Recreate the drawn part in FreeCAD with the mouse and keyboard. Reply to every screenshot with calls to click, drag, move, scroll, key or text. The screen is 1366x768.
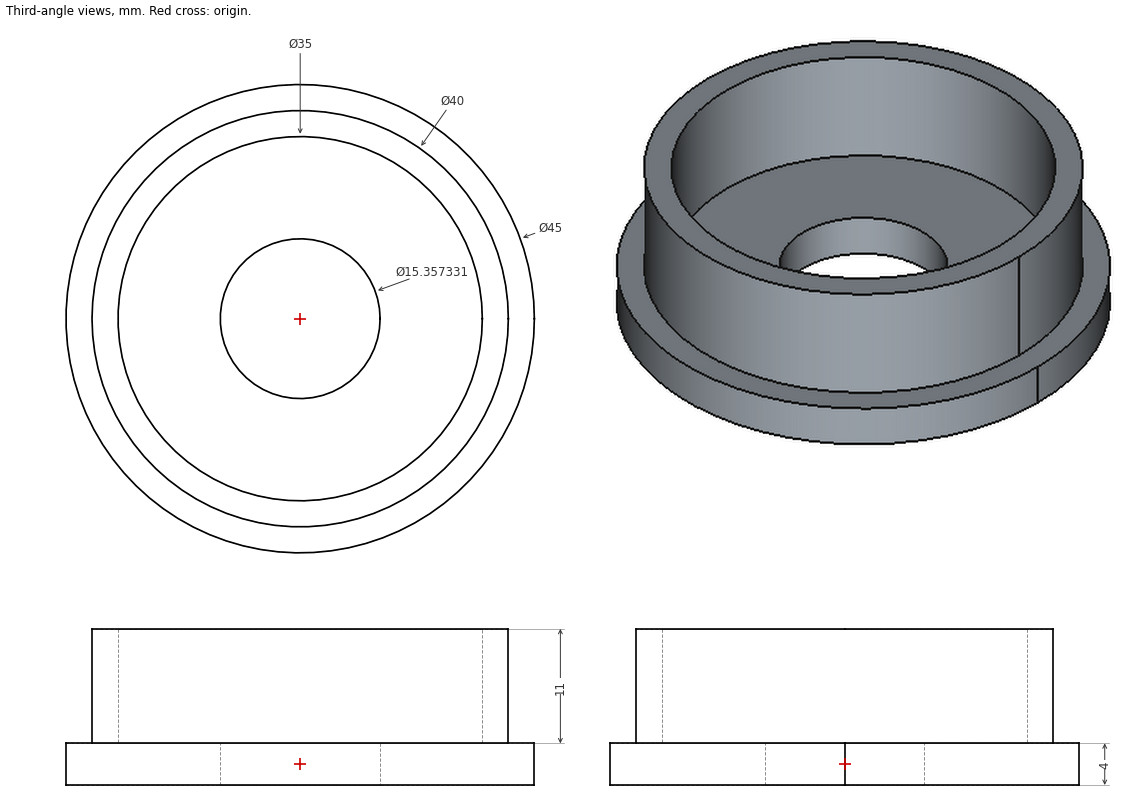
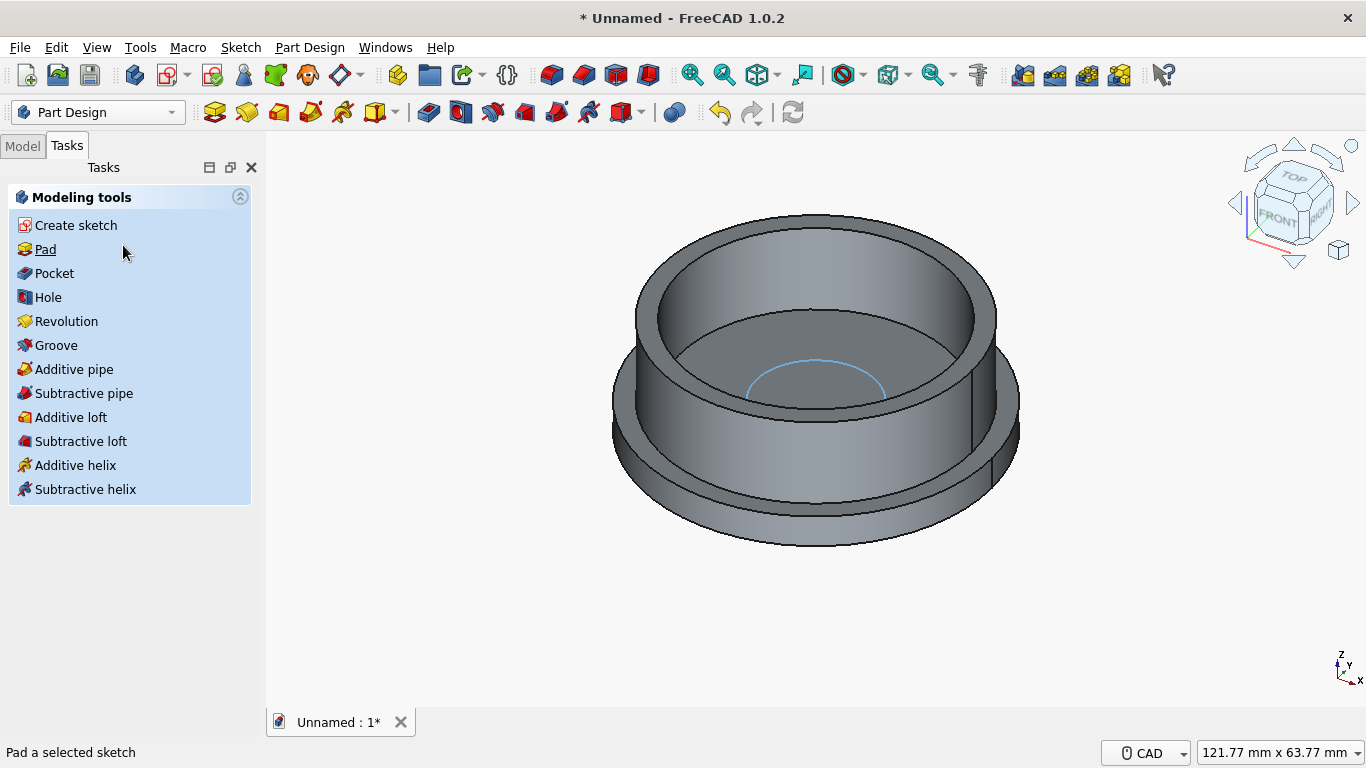
click(430, 112)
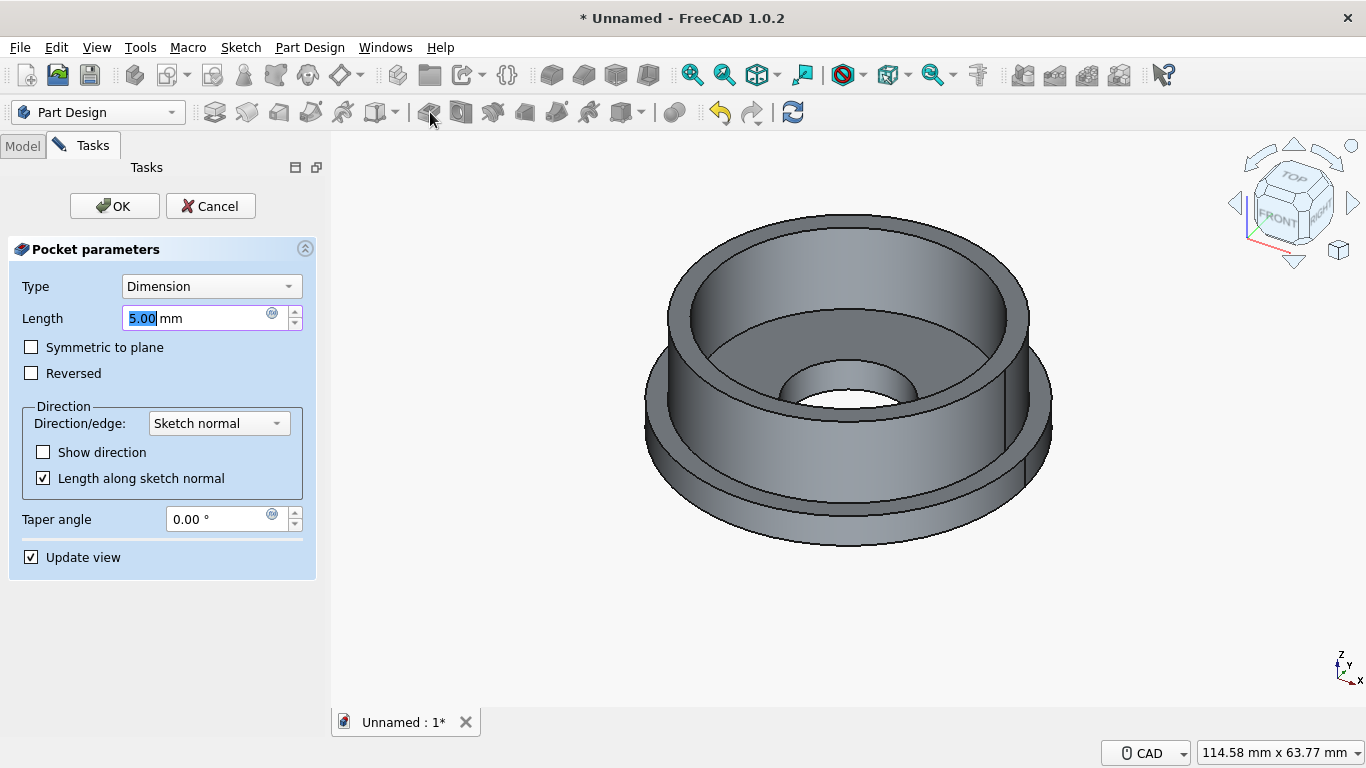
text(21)
key(Tab)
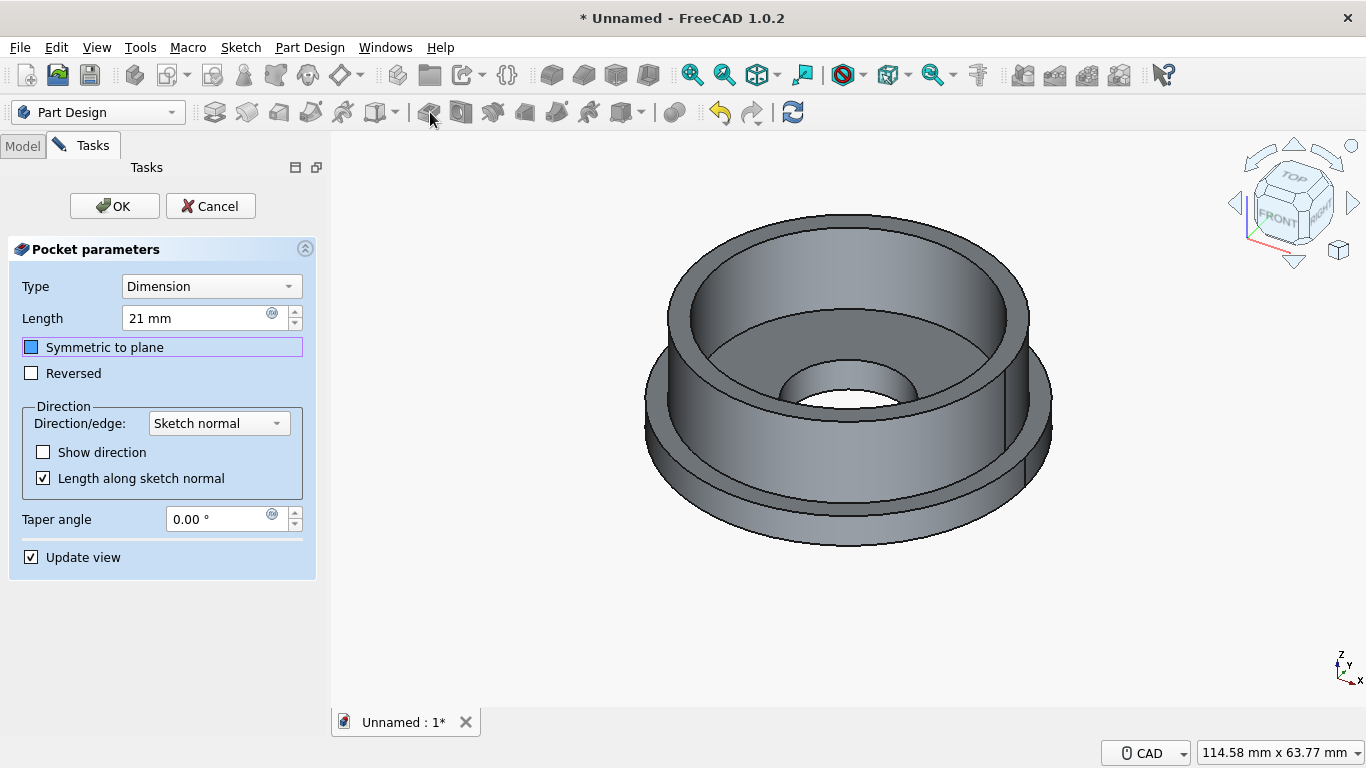
click(115, 206)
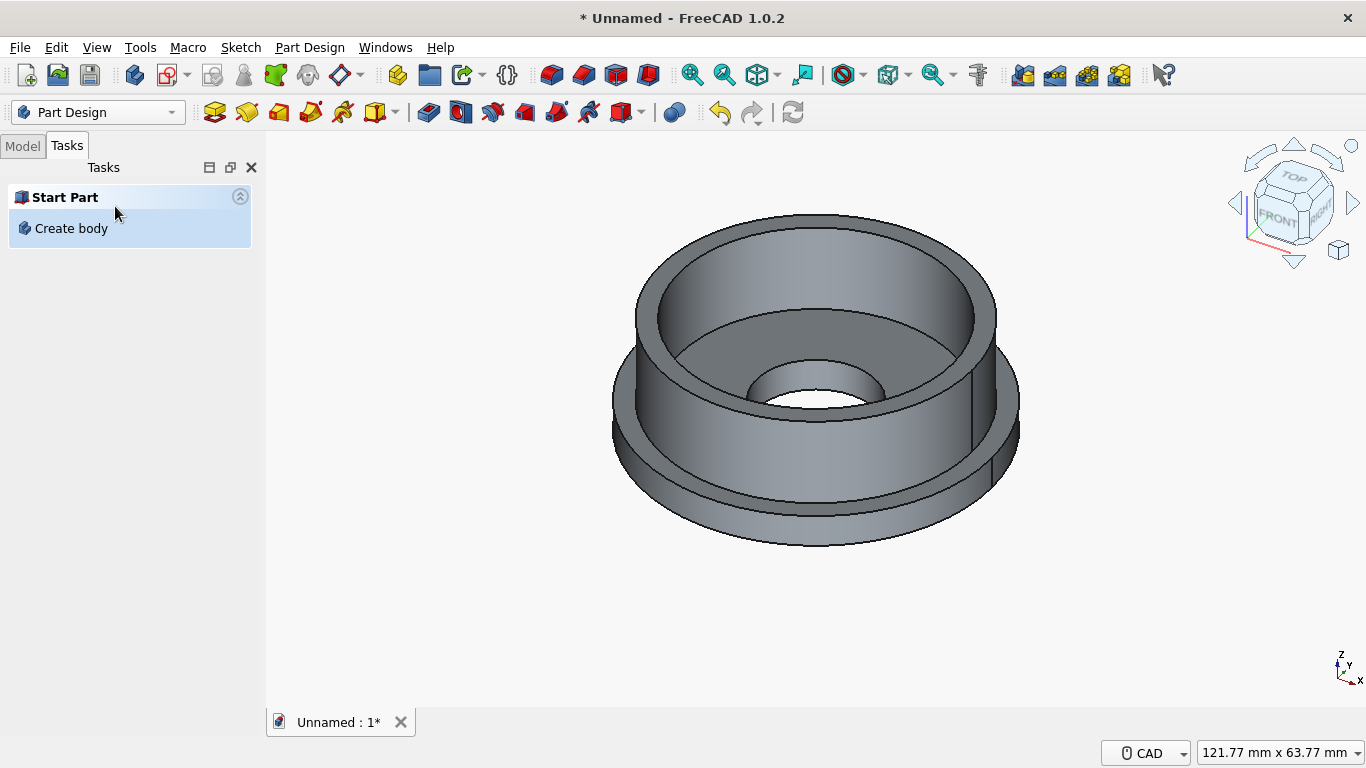
key(0)